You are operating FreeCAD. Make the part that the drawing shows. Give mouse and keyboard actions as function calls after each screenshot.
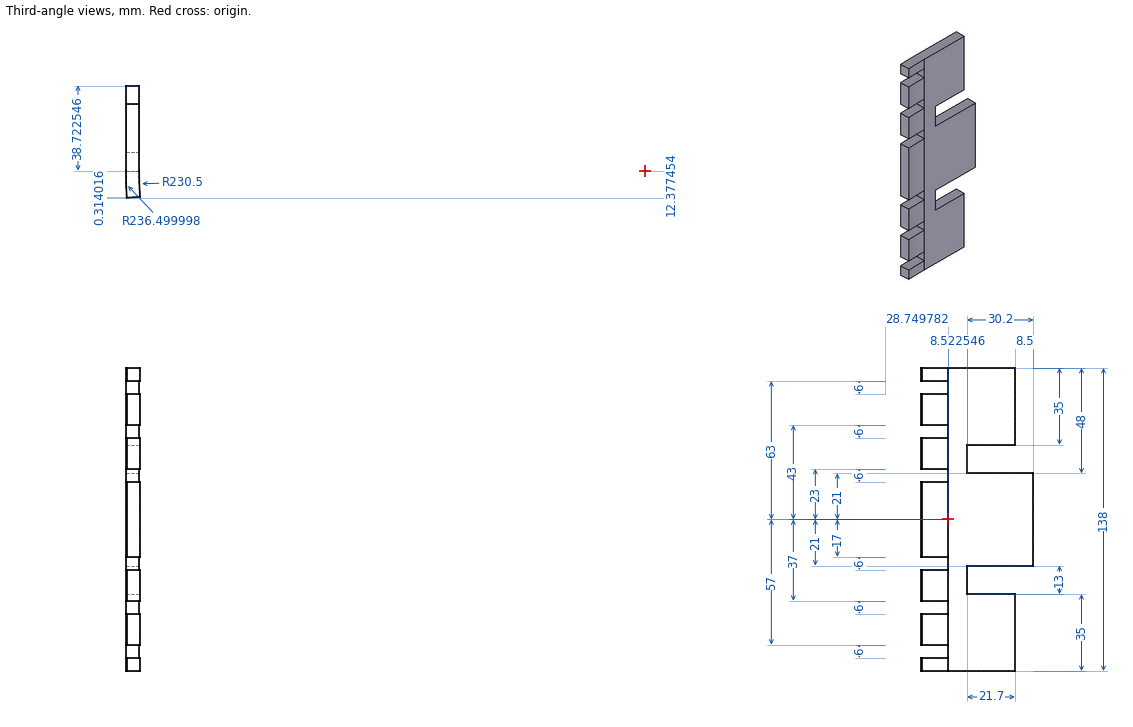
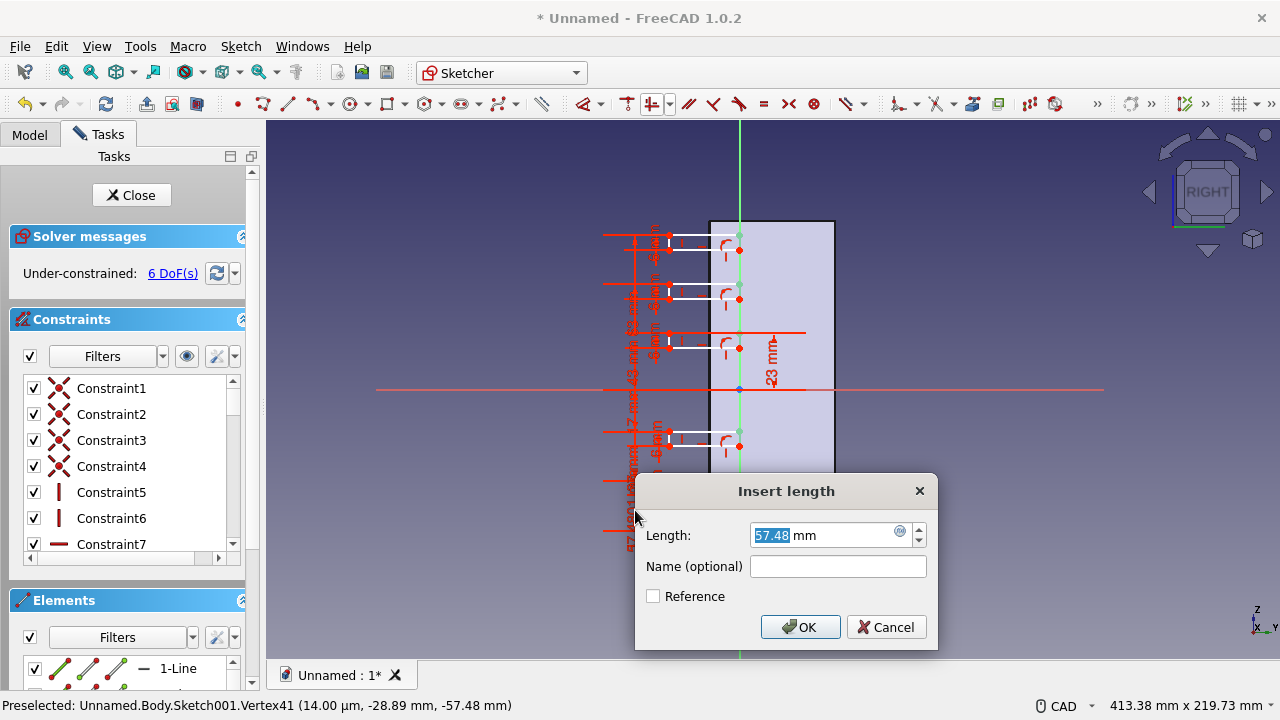
text(57)
key(Return)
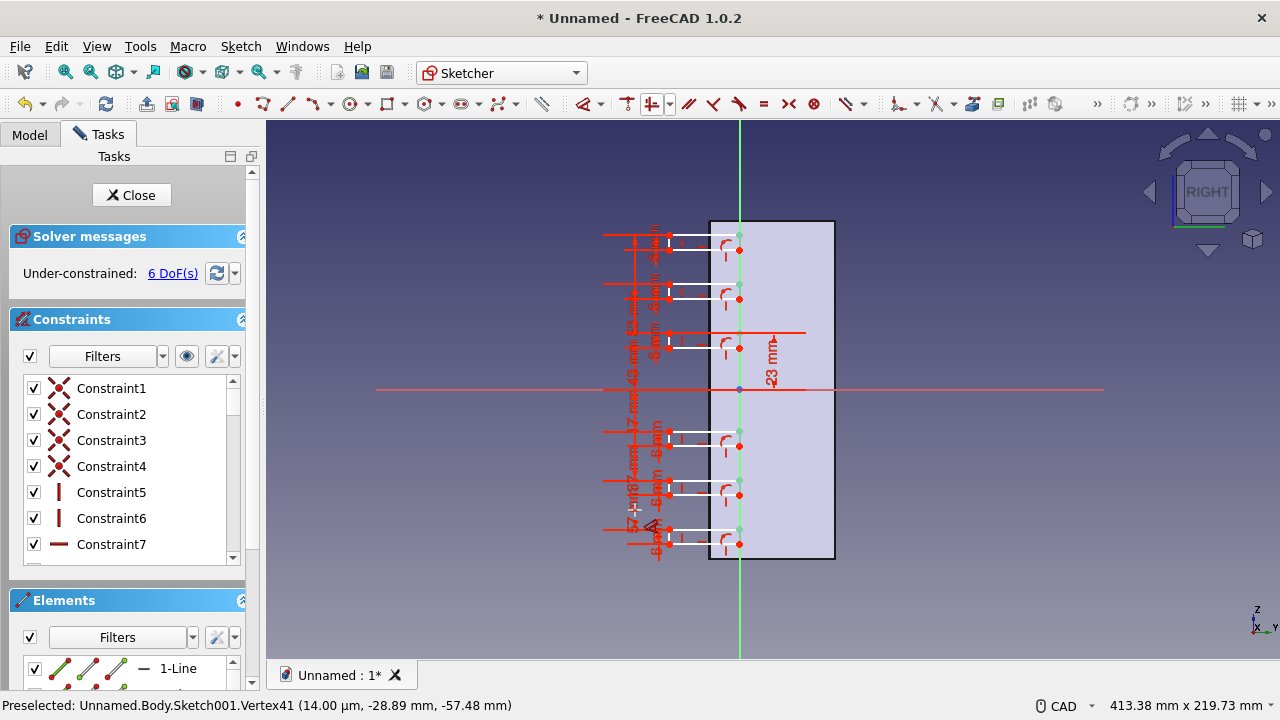
click(690, 250)
click(704, 216)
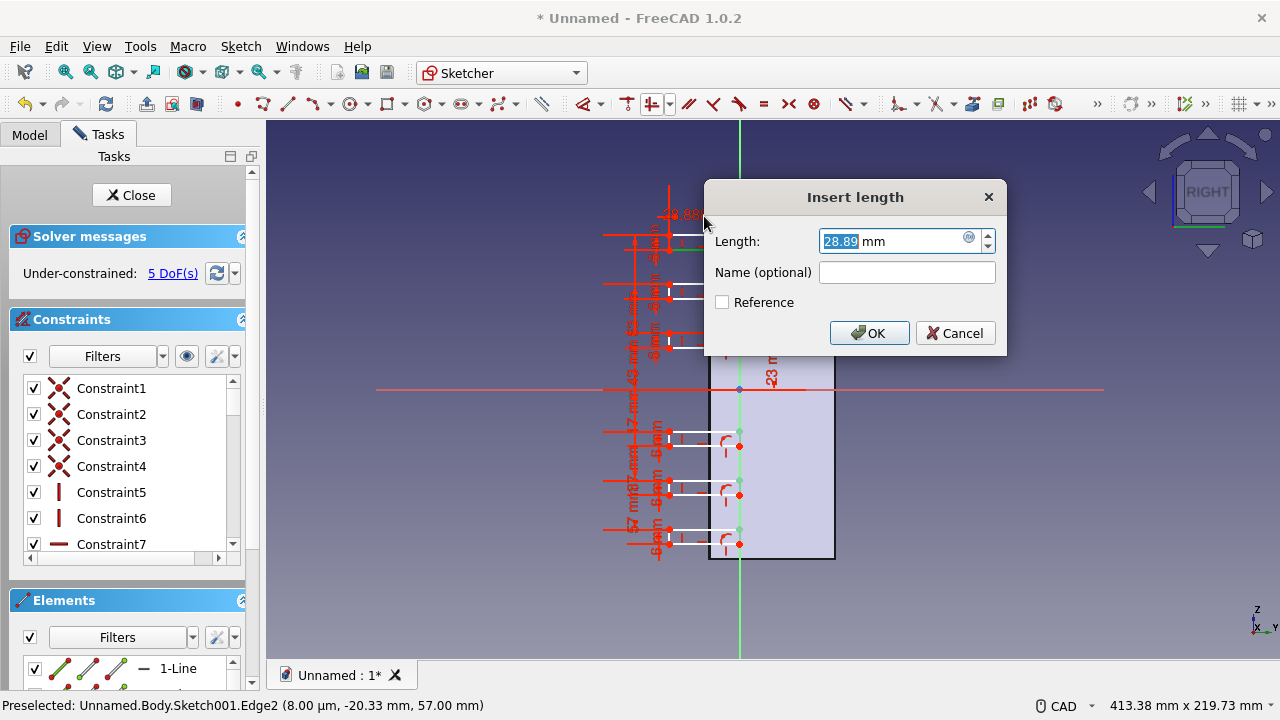
text(28.749782)
key(Return)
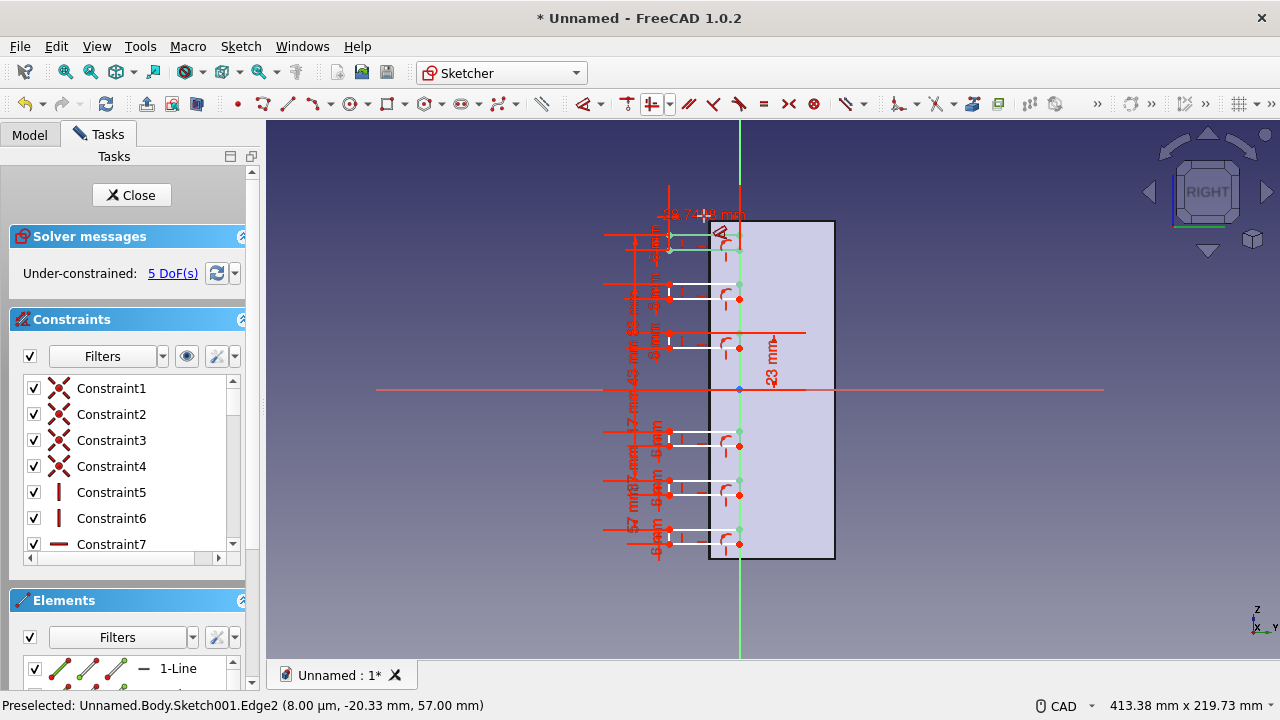
click(690, 299)
click(704, 265)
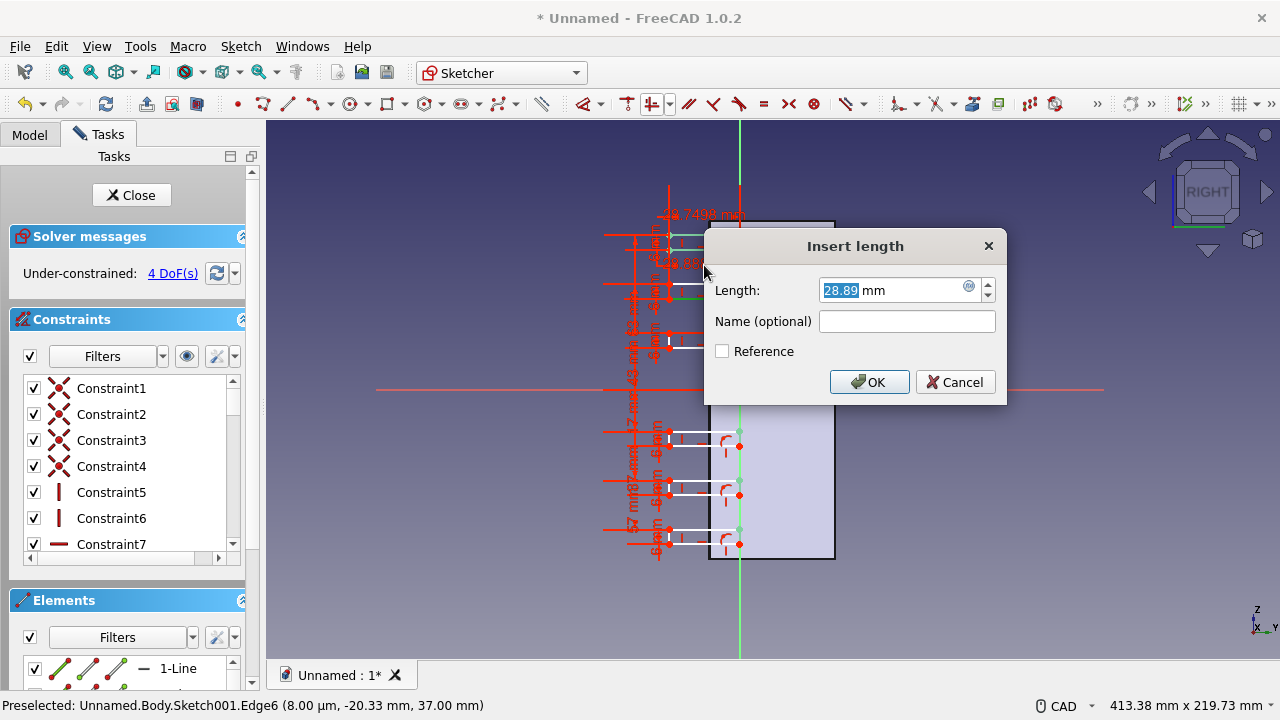
text(28.749782)
key(Return)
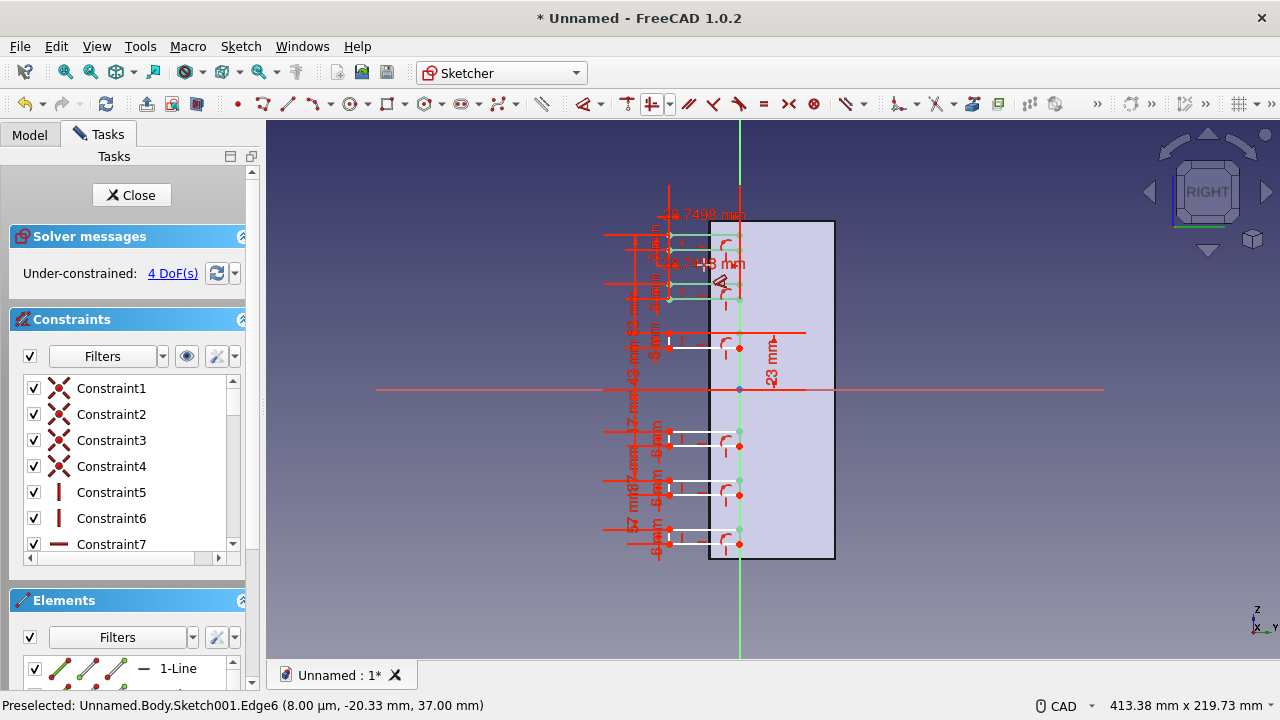
click(690, 348)
click(721, 314)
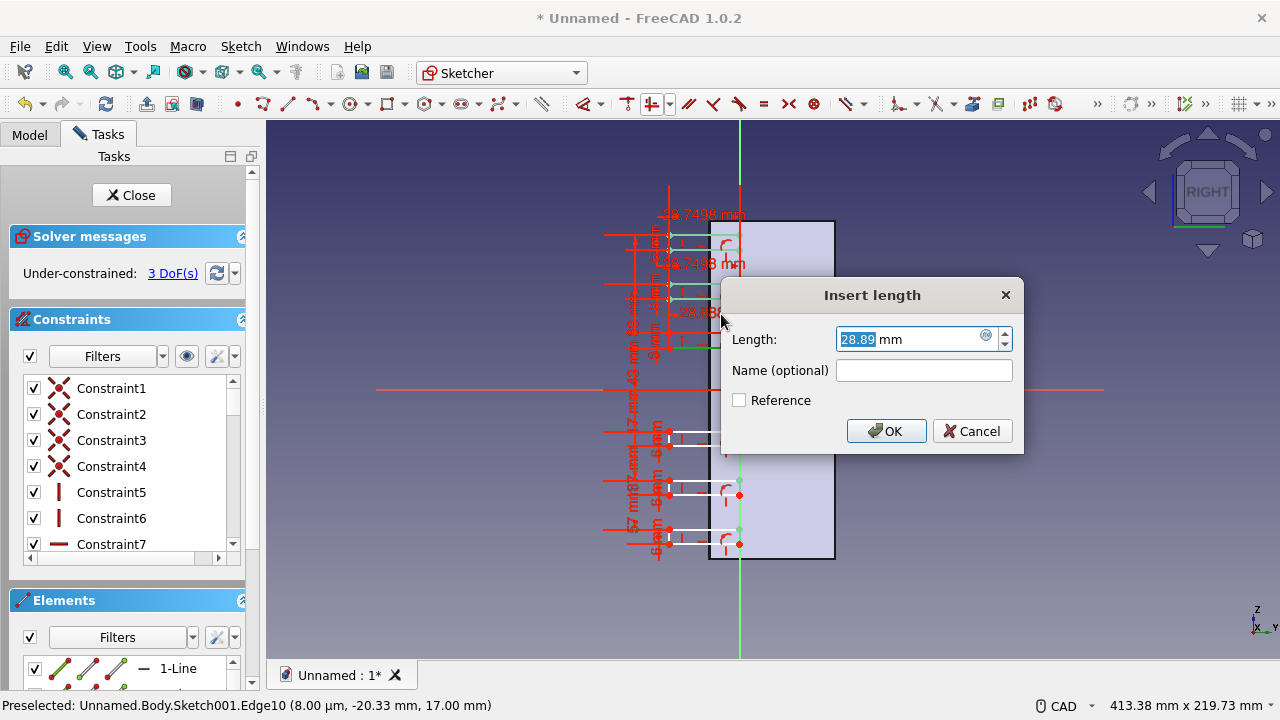
text(28.749782)
key(Return)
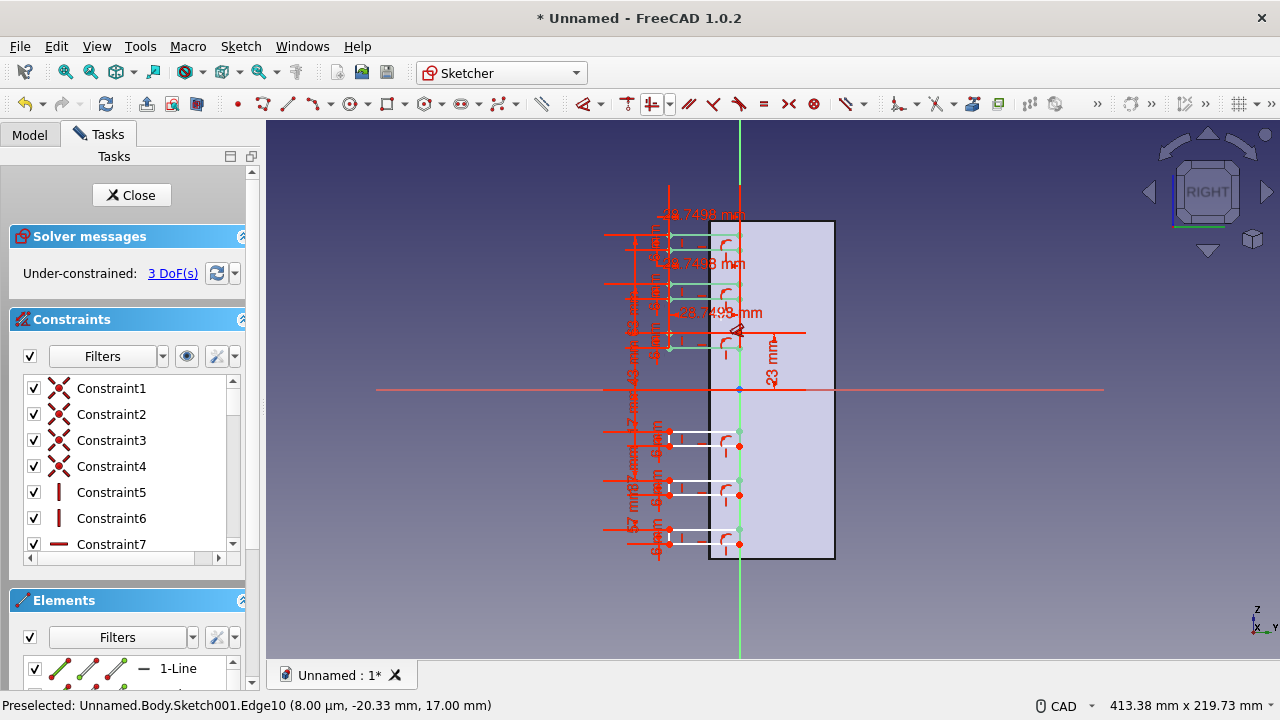
click(690, 446)
click(721, 412)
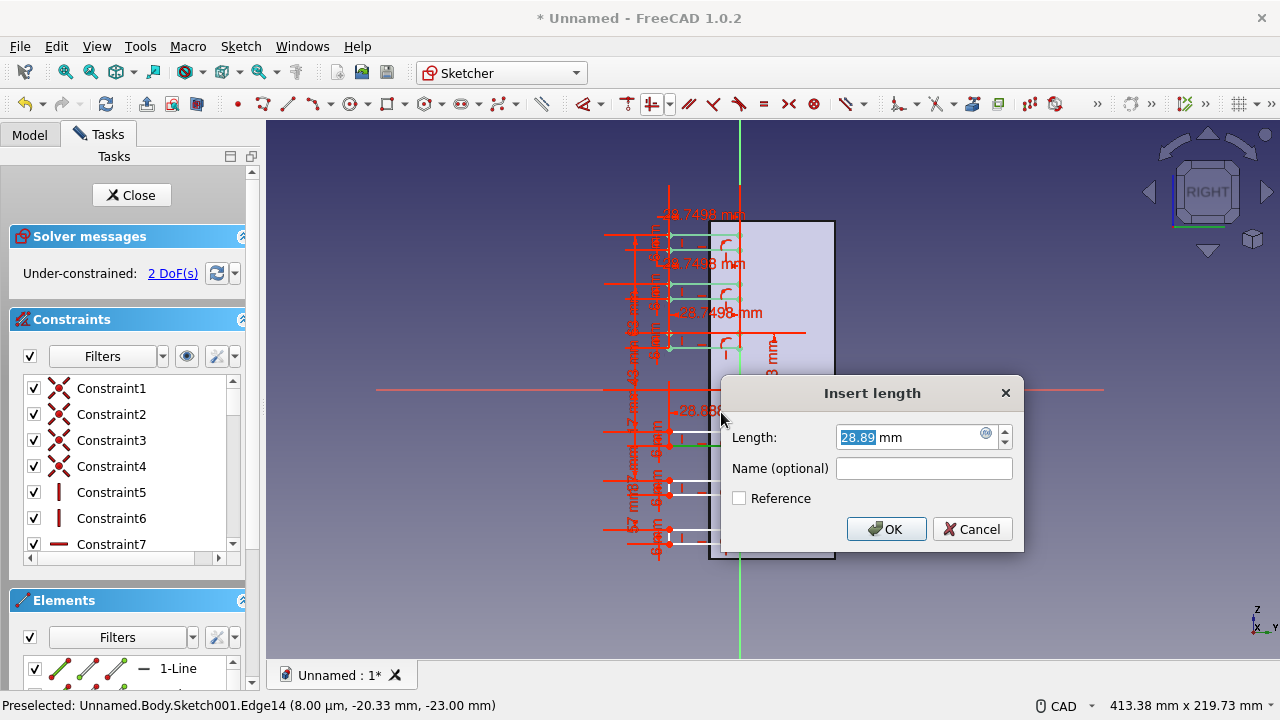
text(28.749782)
key(Return)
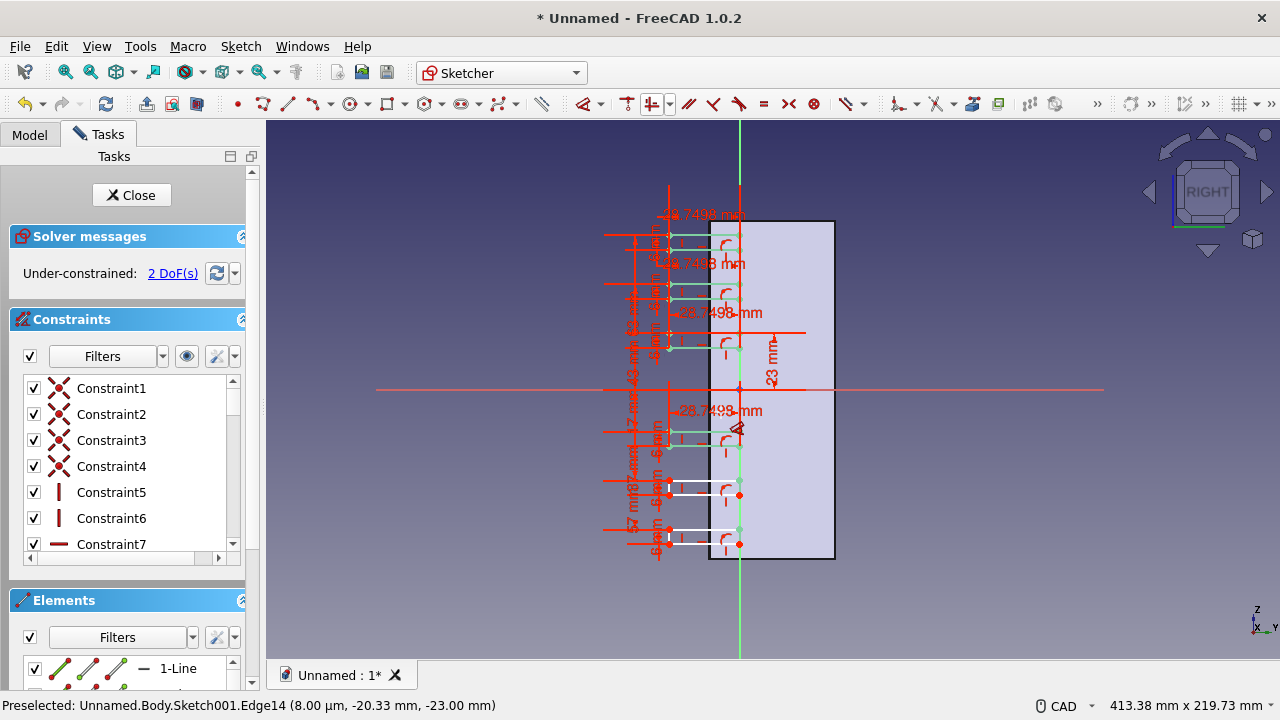
click(690, 495)
click(721, 461)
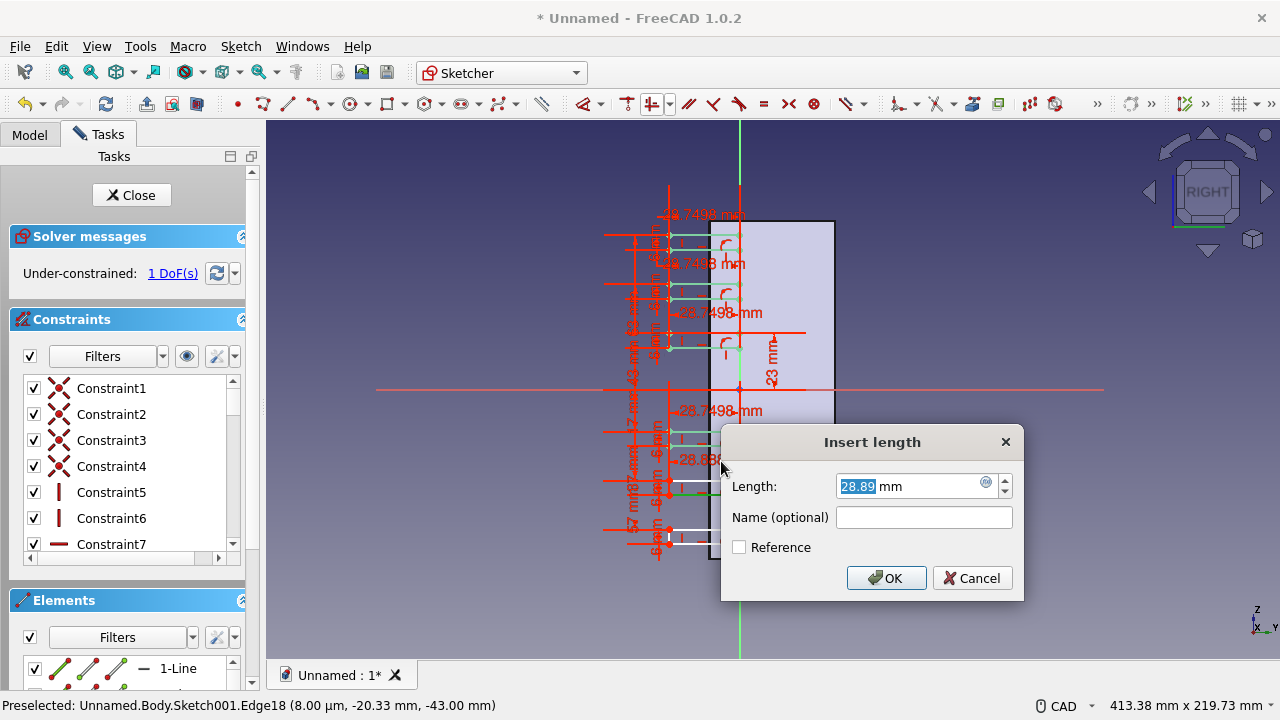
text(28.749782)
key(Return)